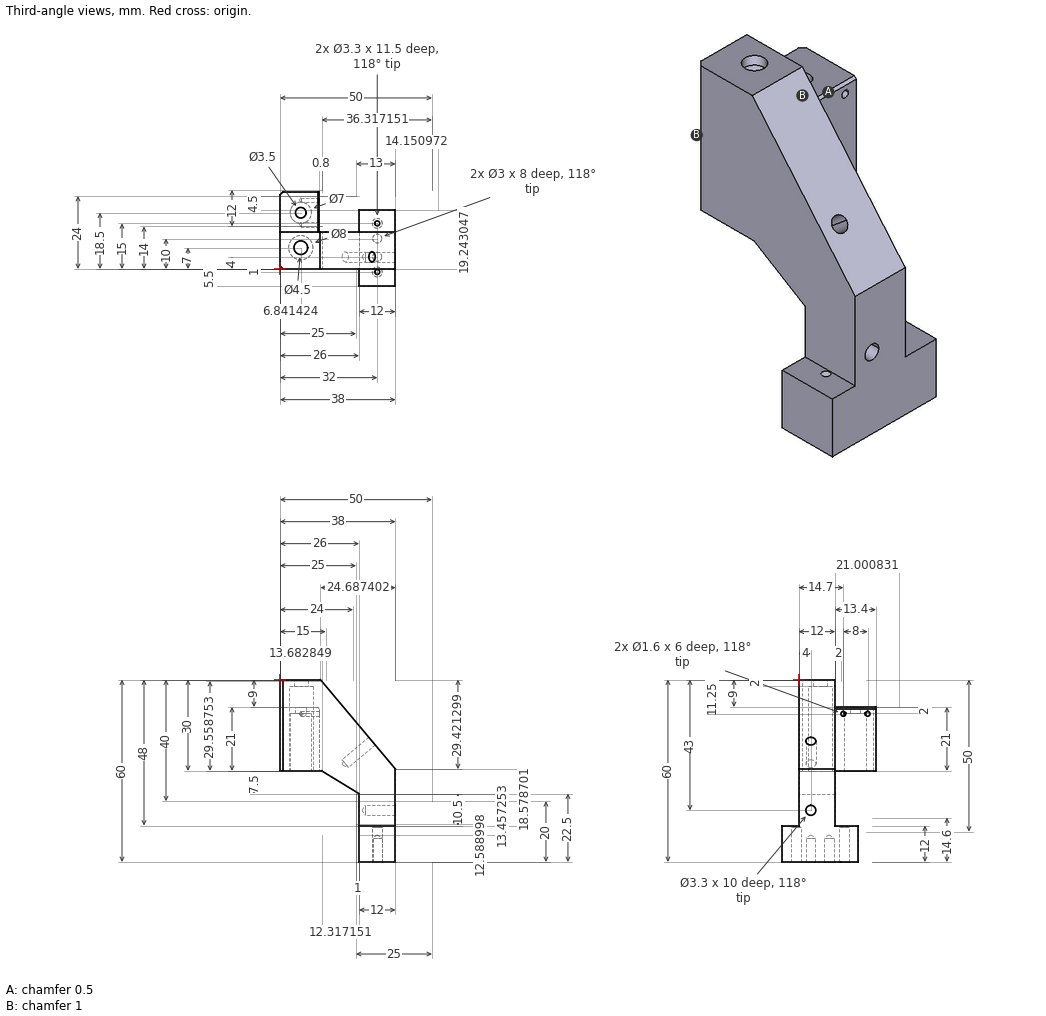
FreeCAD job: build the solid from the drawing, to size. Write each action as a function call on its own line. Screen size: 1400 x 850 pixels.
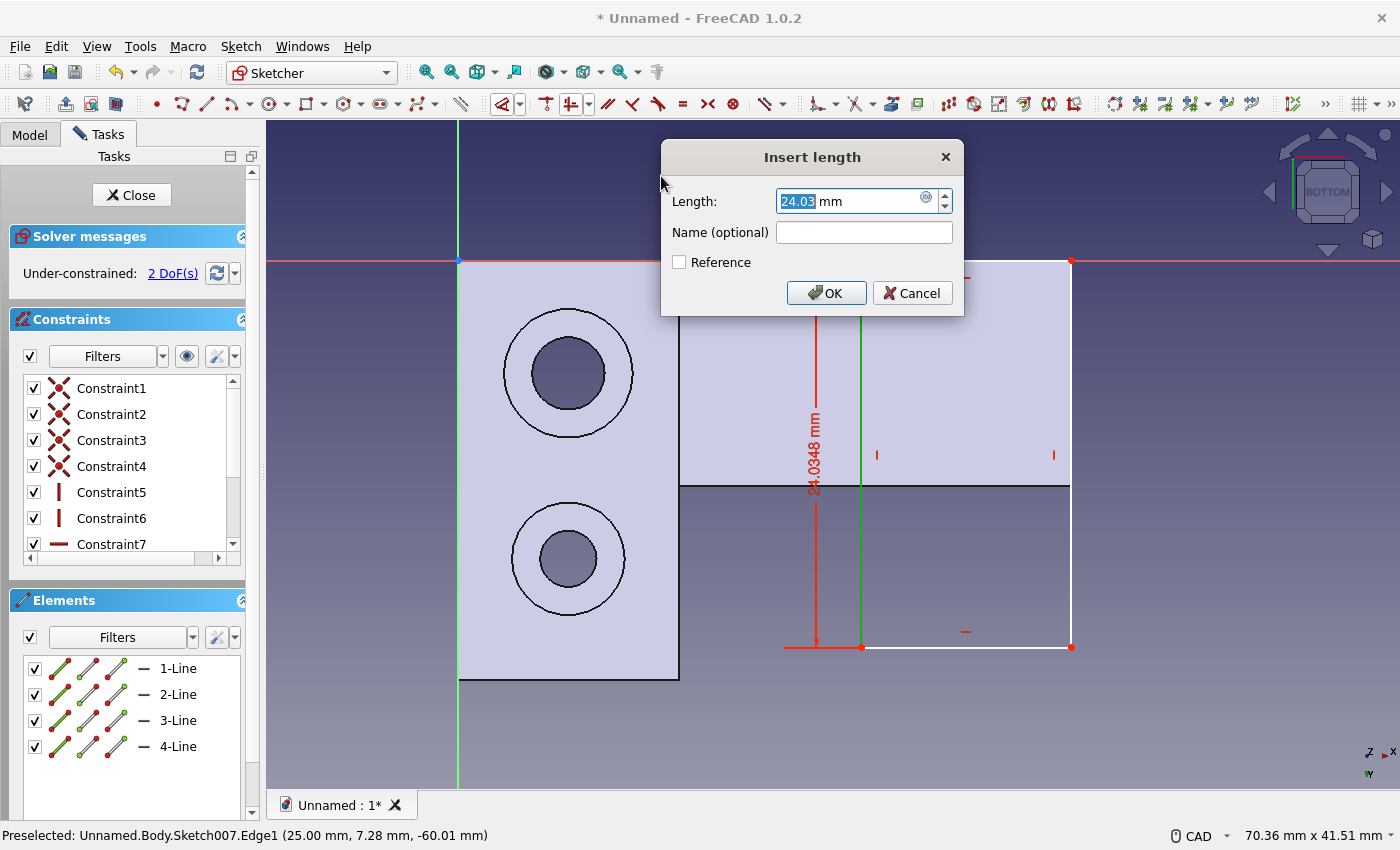
text(24)
key(Return)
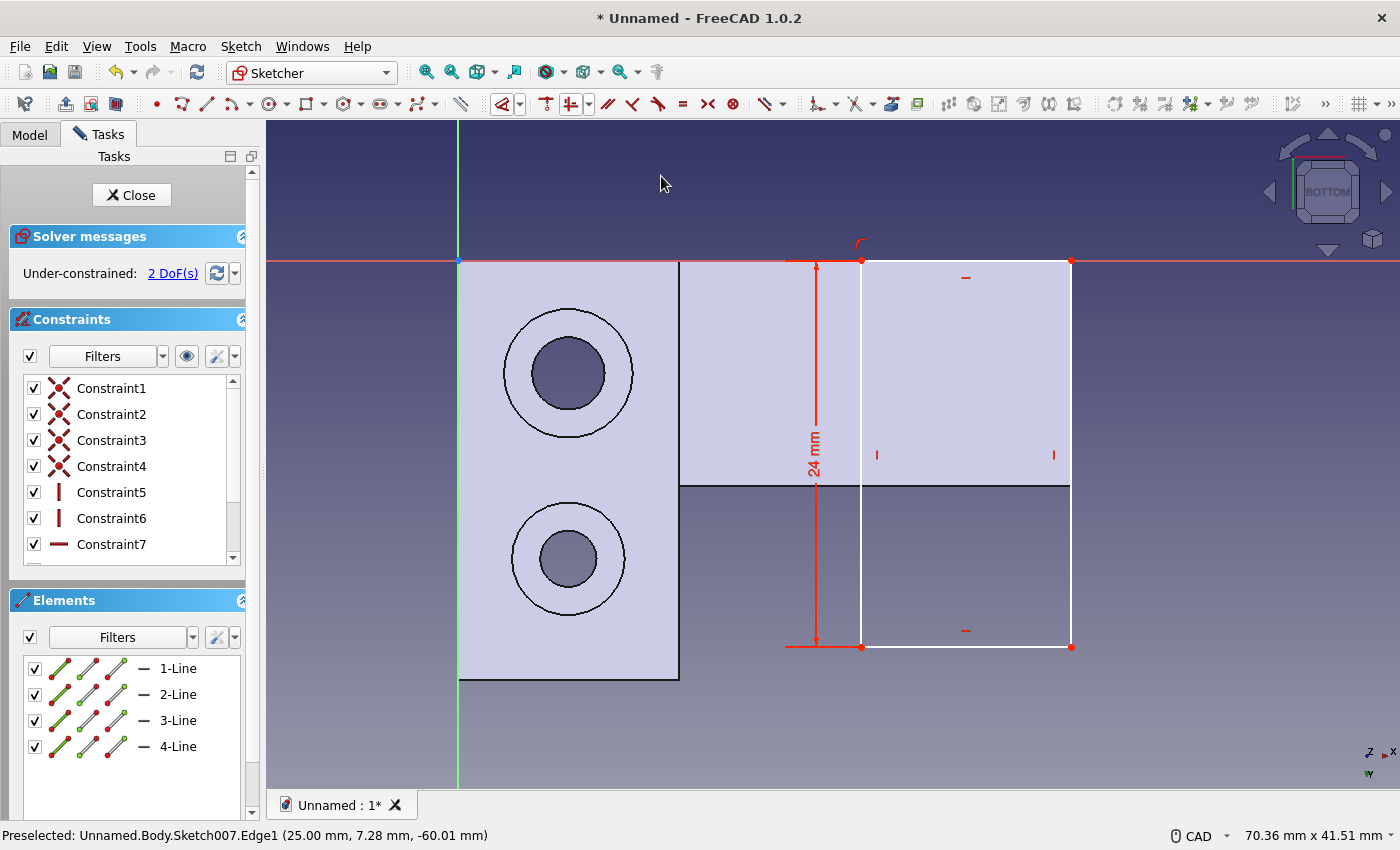
click(924, 647)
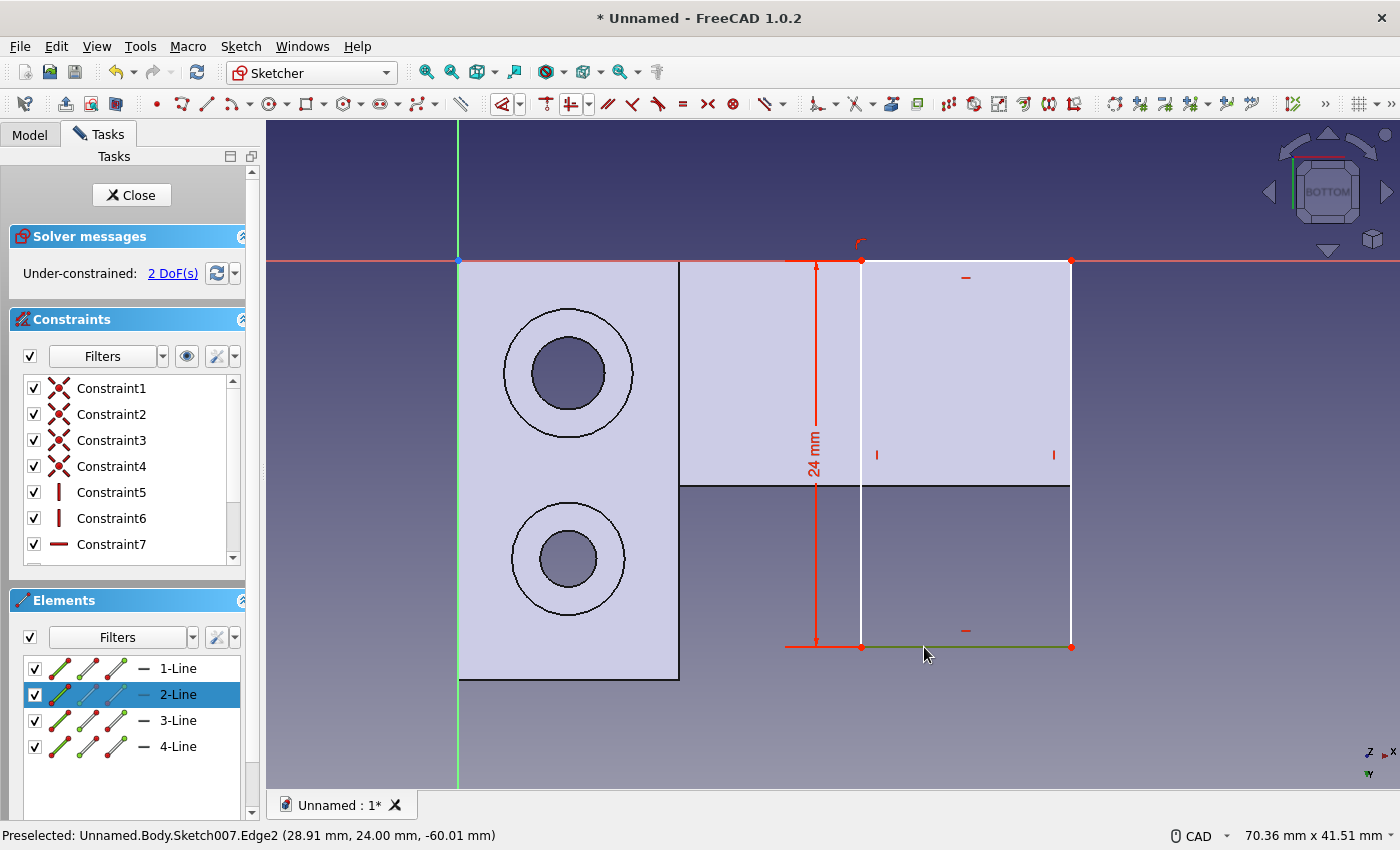
click(520, 104)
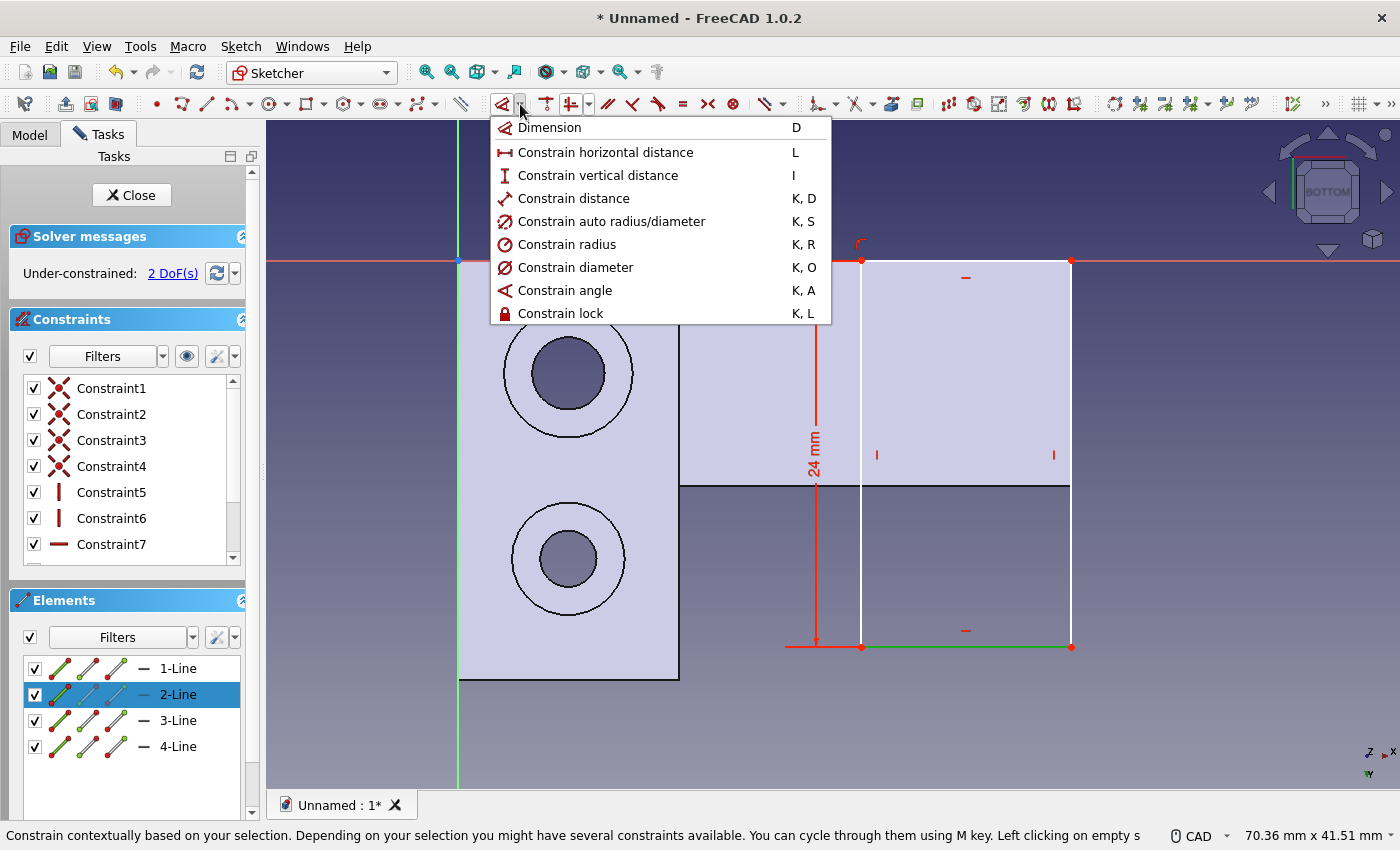
click(661, 152)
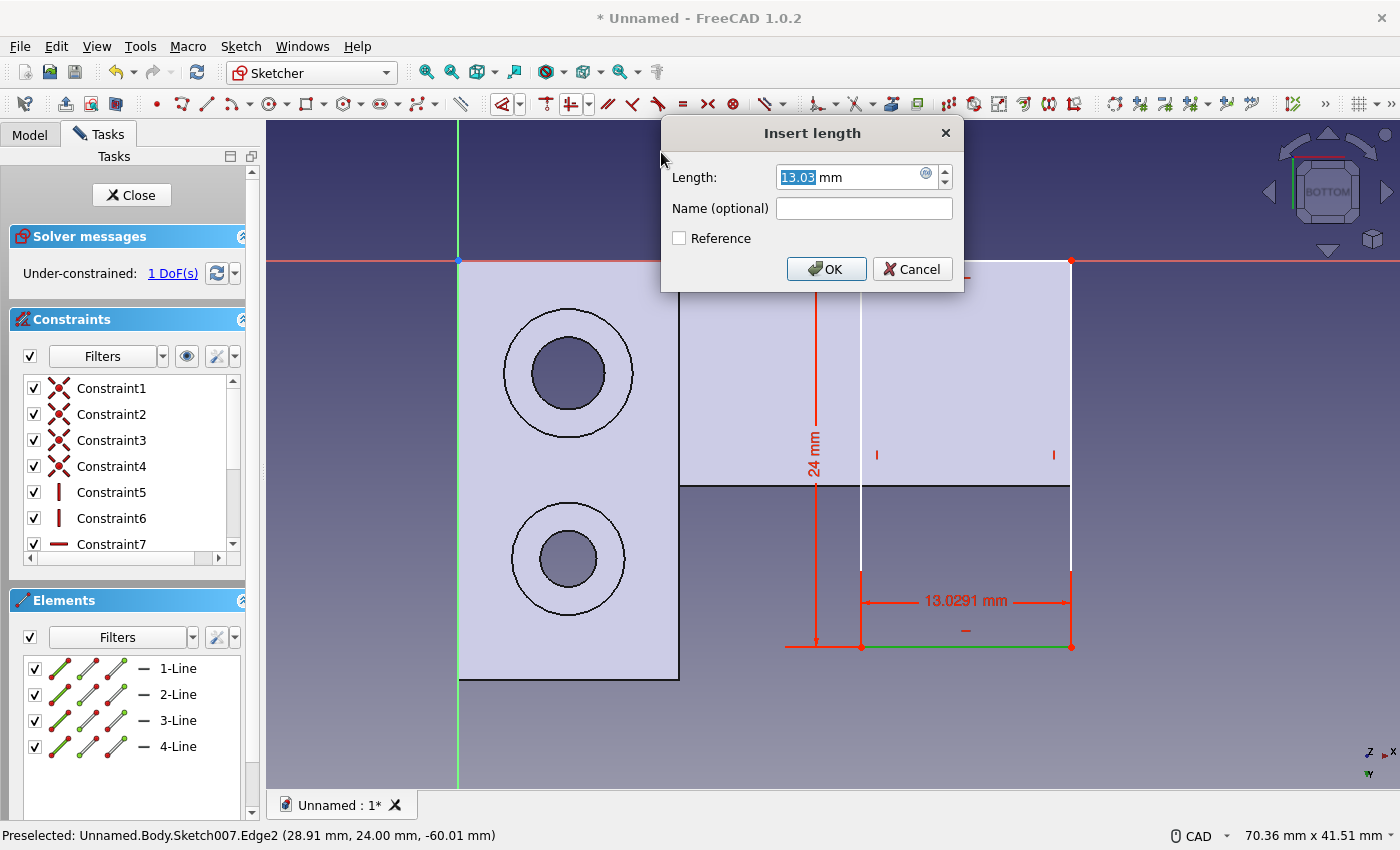
text(13)
key(Return)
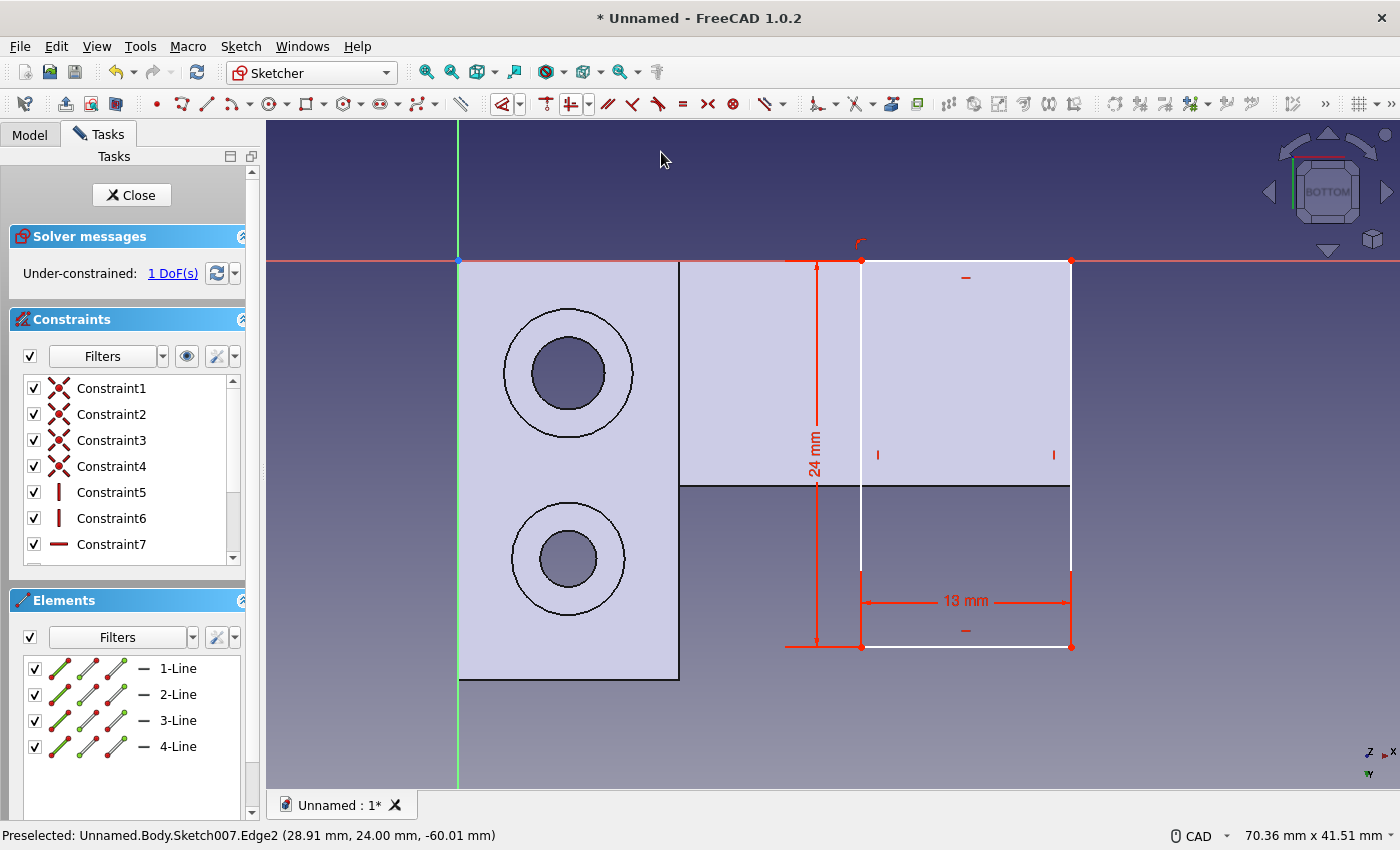
click(861, 261)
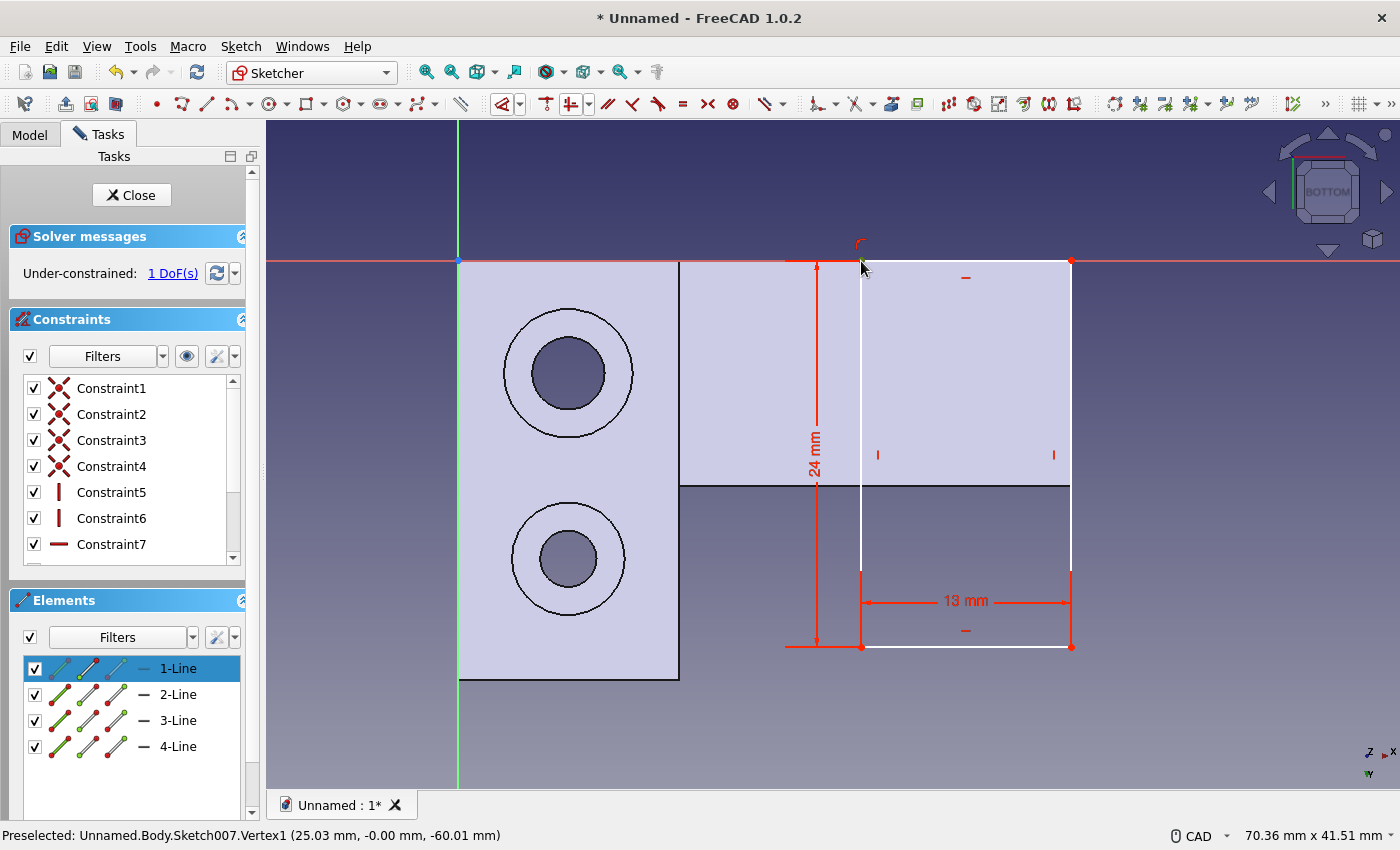
key(l)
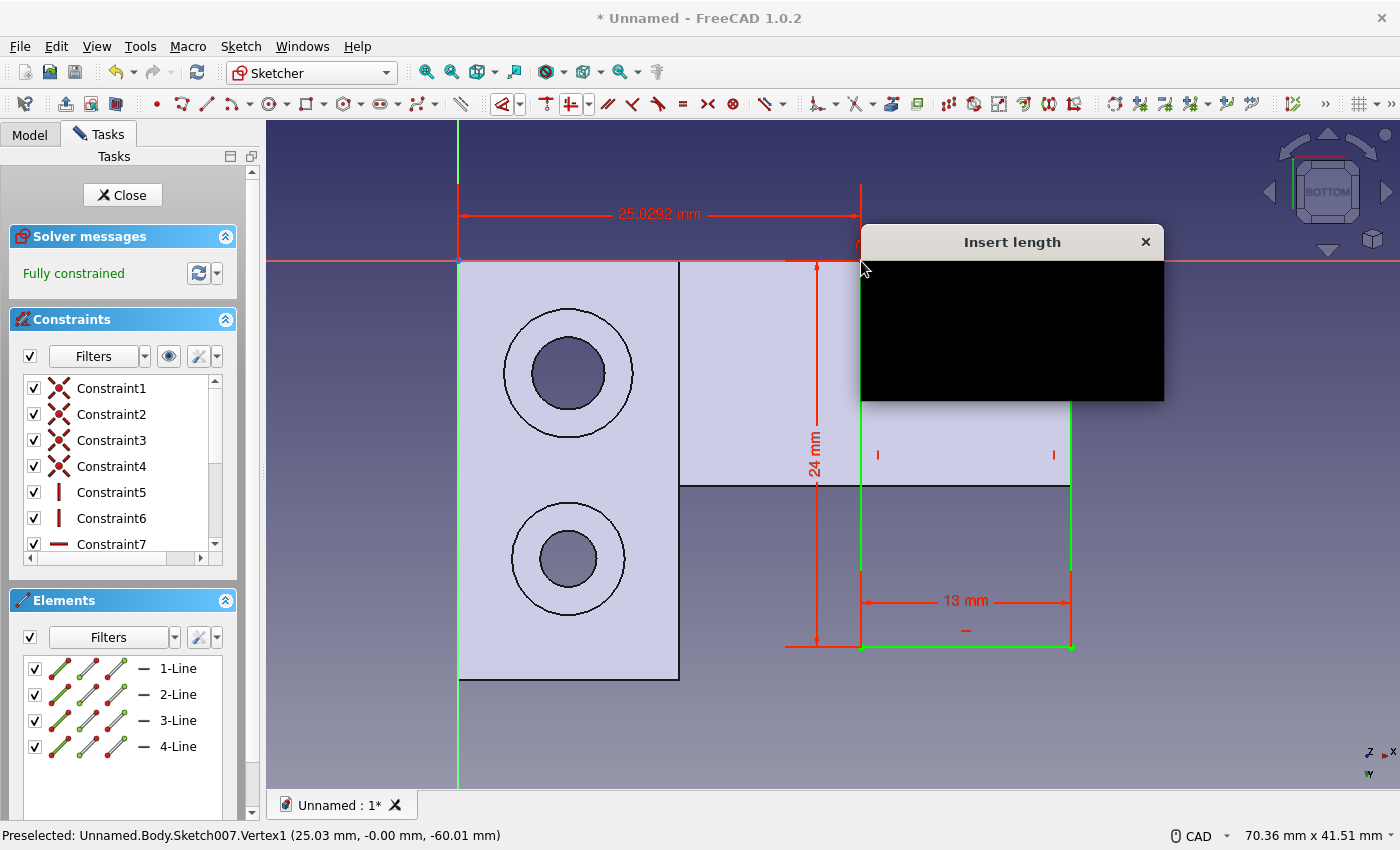
text(25)
key(Return)